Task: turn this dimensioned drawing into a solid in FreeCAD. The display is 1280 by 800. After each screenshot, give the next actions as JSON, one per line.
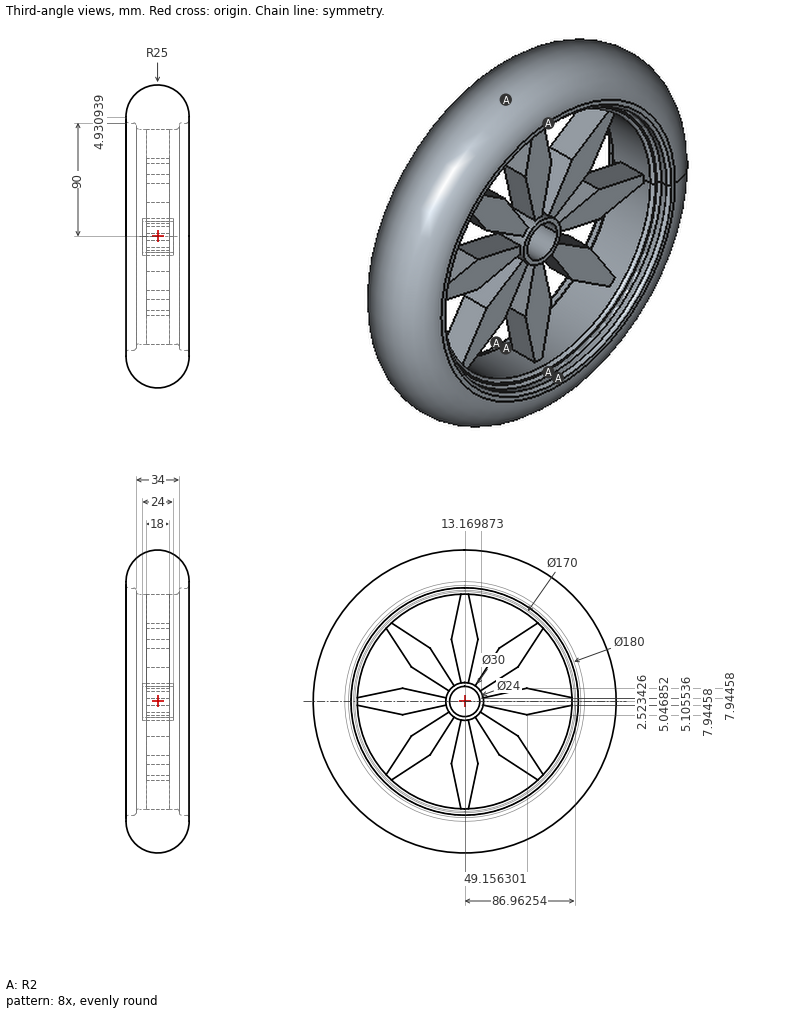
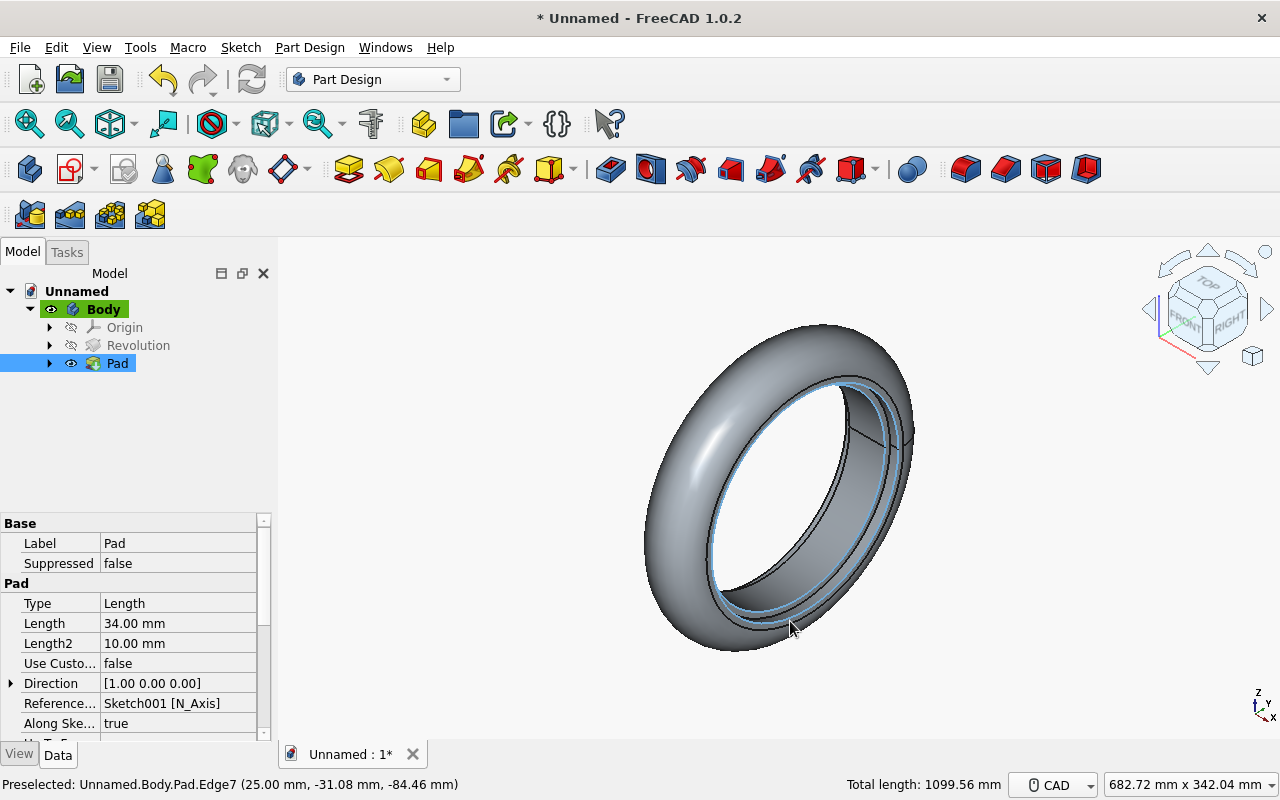
{"action": "key", "text": "2"}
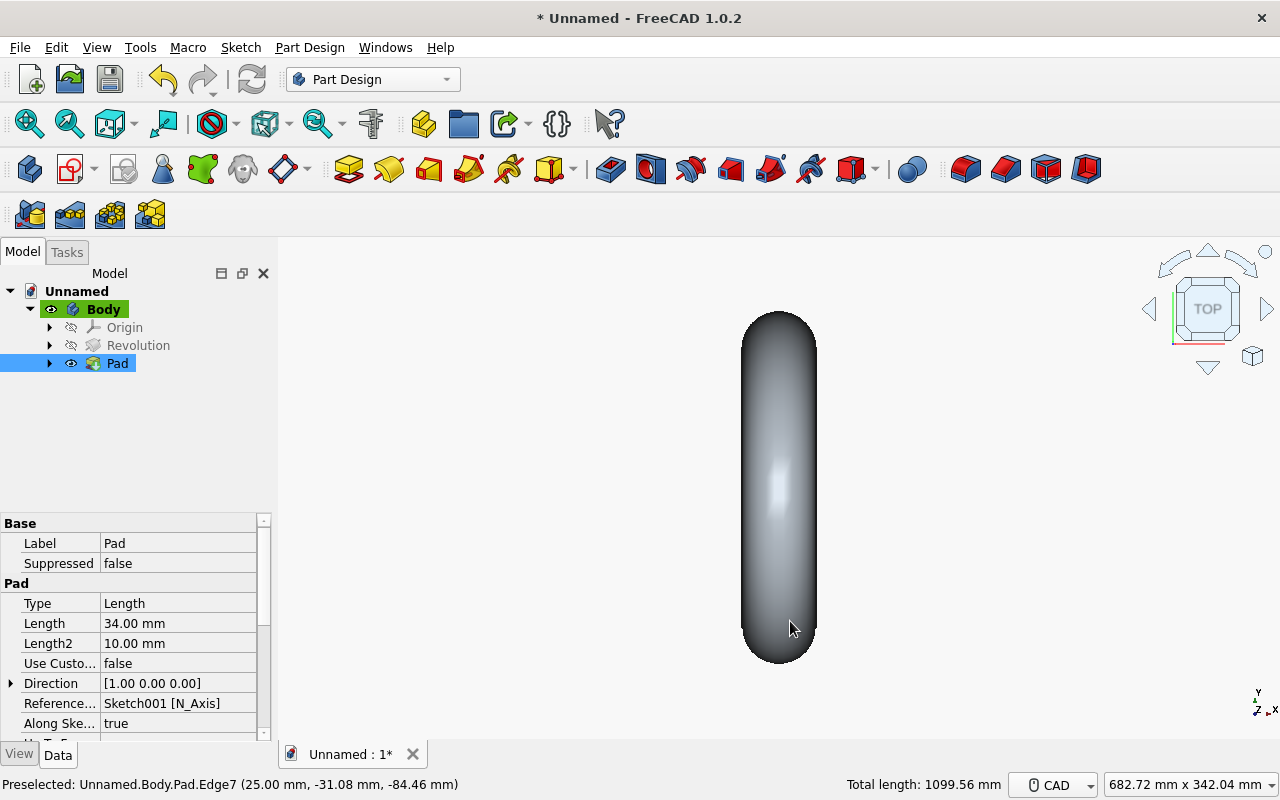
{"action": "key", "text": "1"}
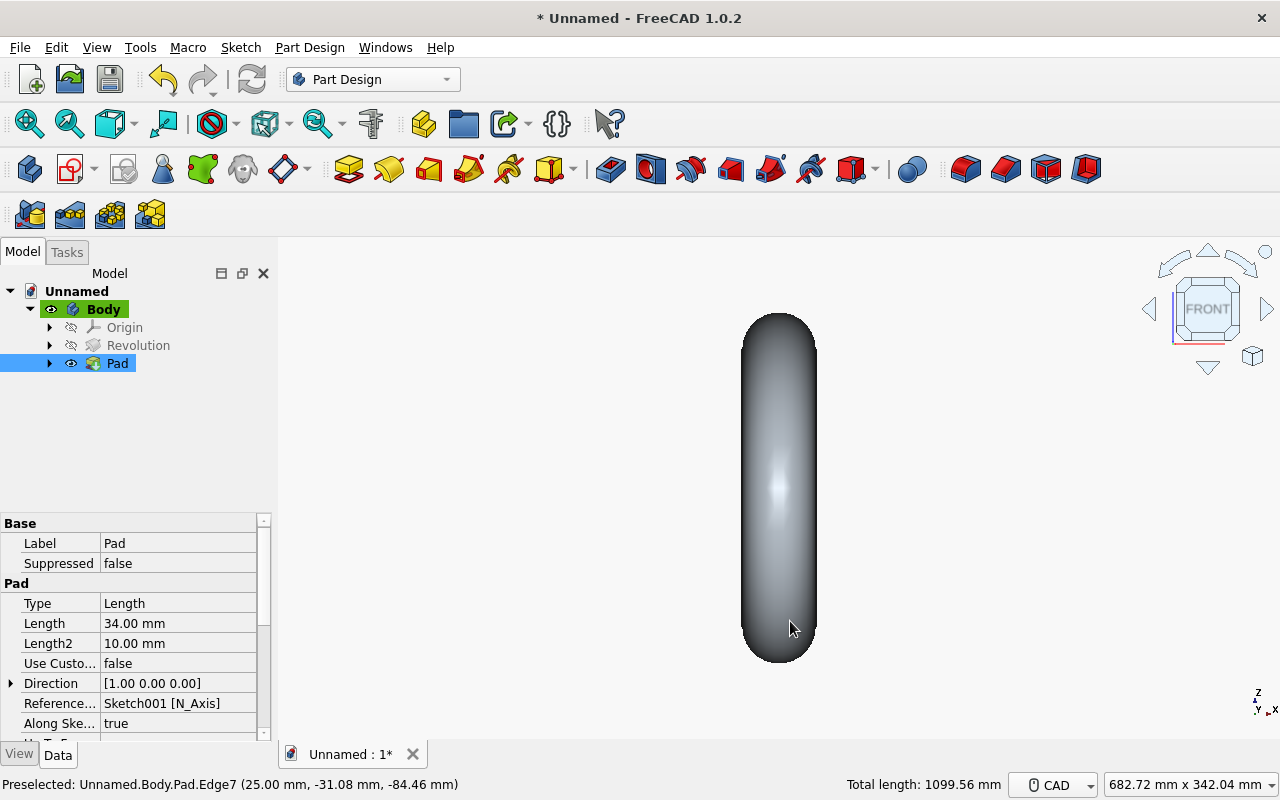
{"action": "key", "text": "3"}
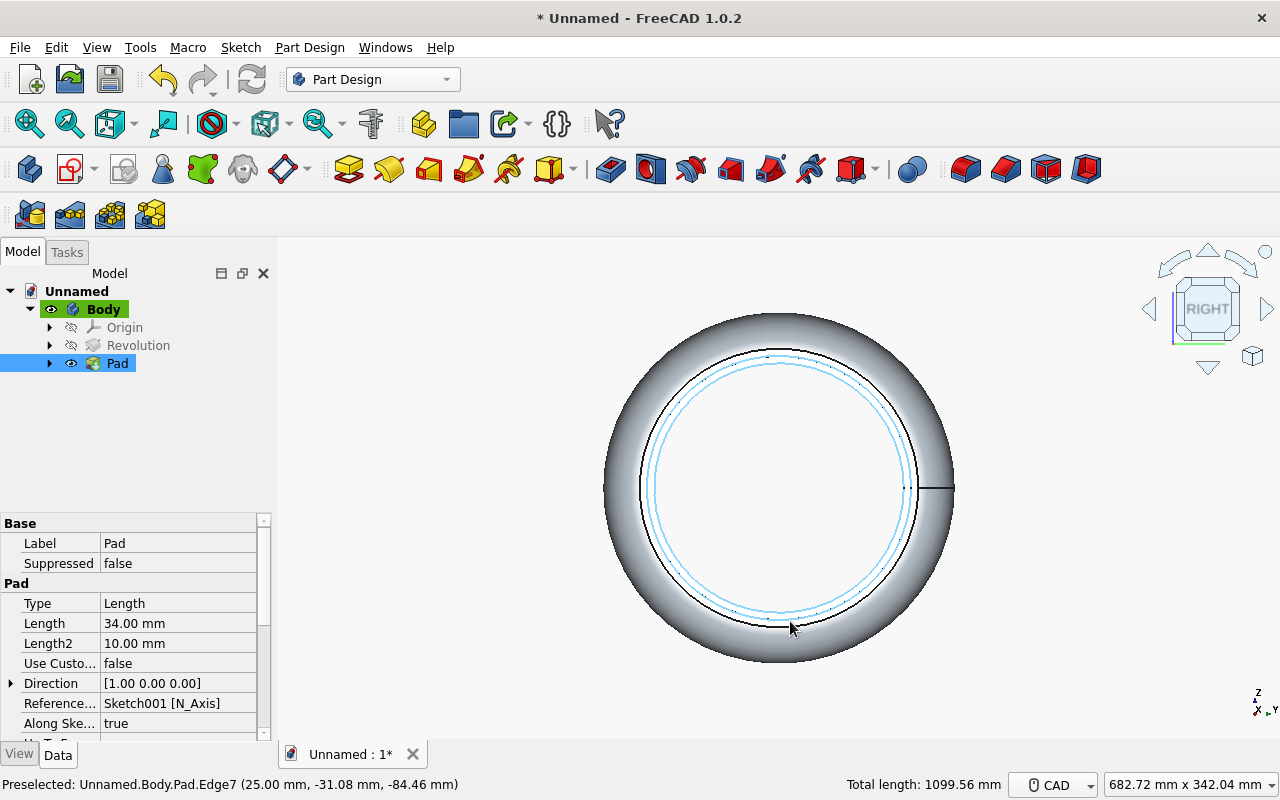
{"action": "key", "text": "5"}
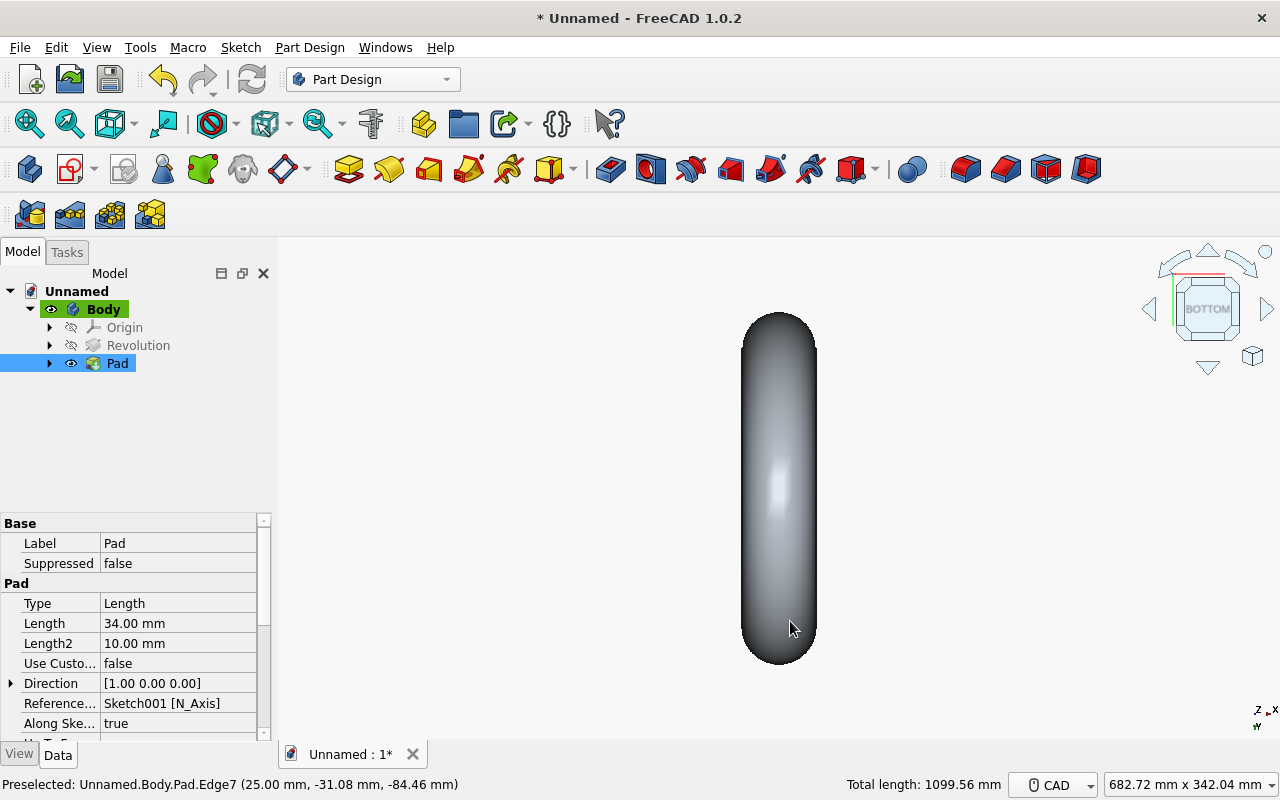
{"action": "key", "text": "4"}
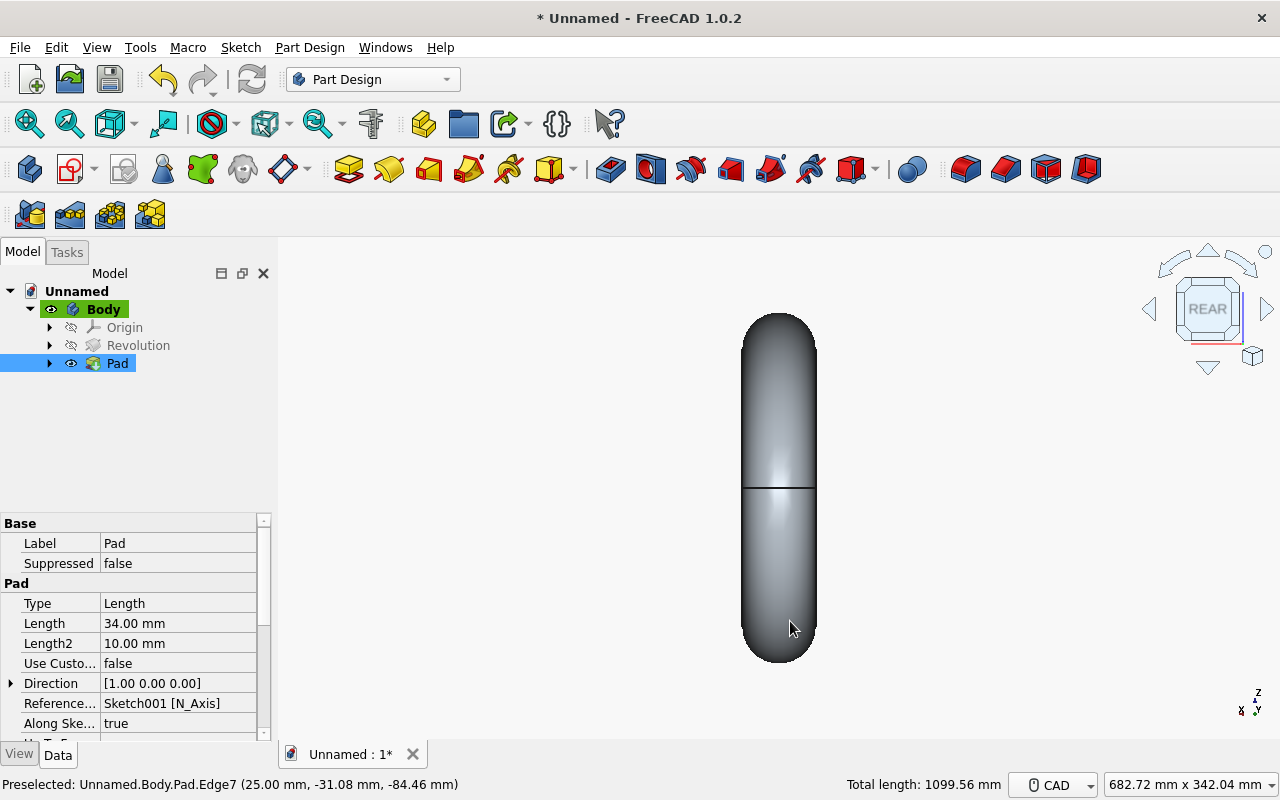
{"action": "key", "text": "6"}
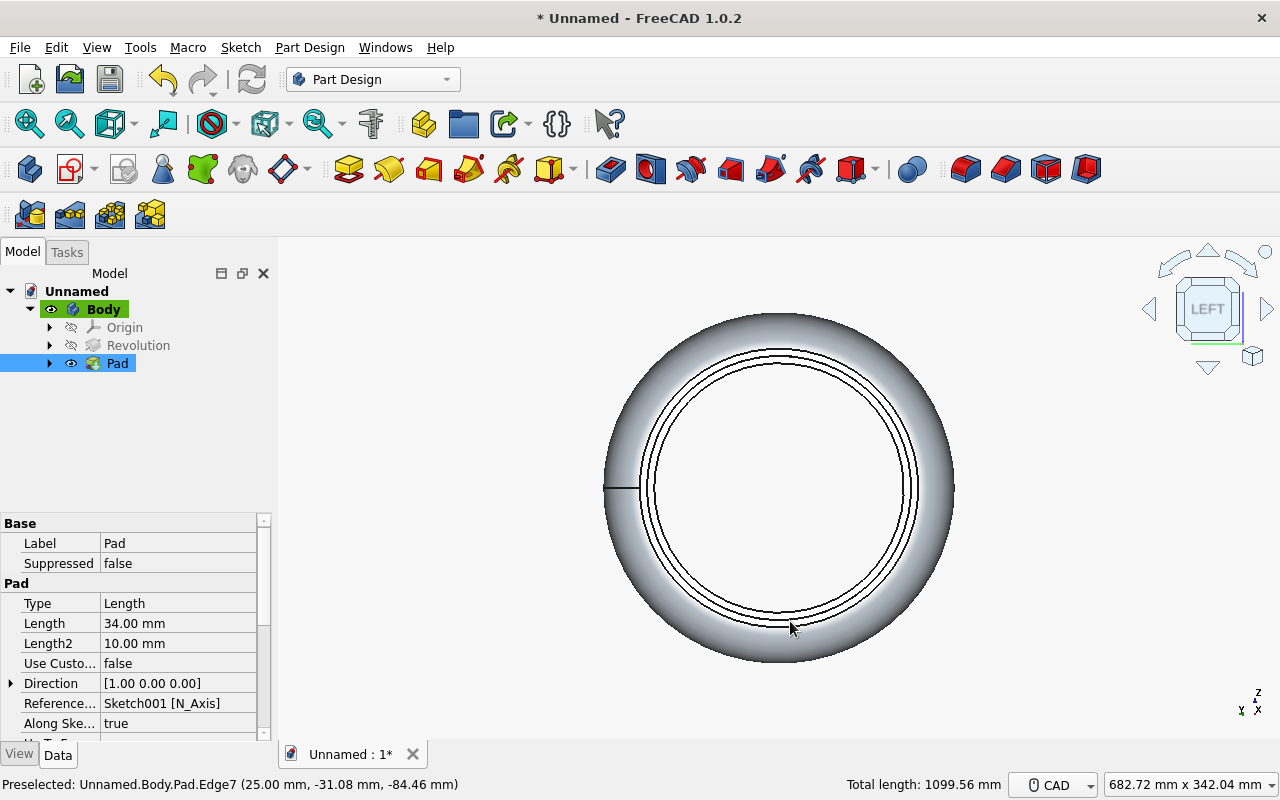
{"action": "left_click", "coordinate": [904, 487], "text": "ctrl"}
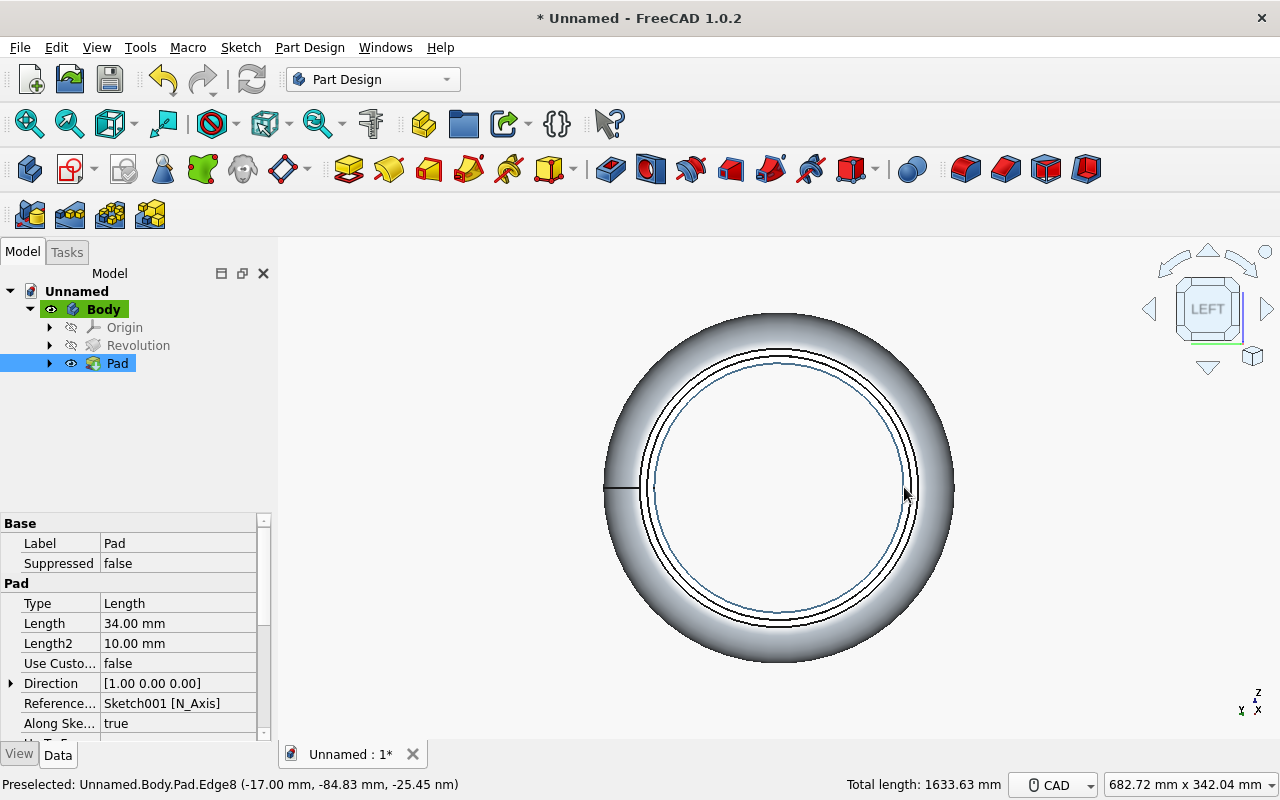
{"action": "left_click", "coordinate": [911, 487], "text": "ctrl"}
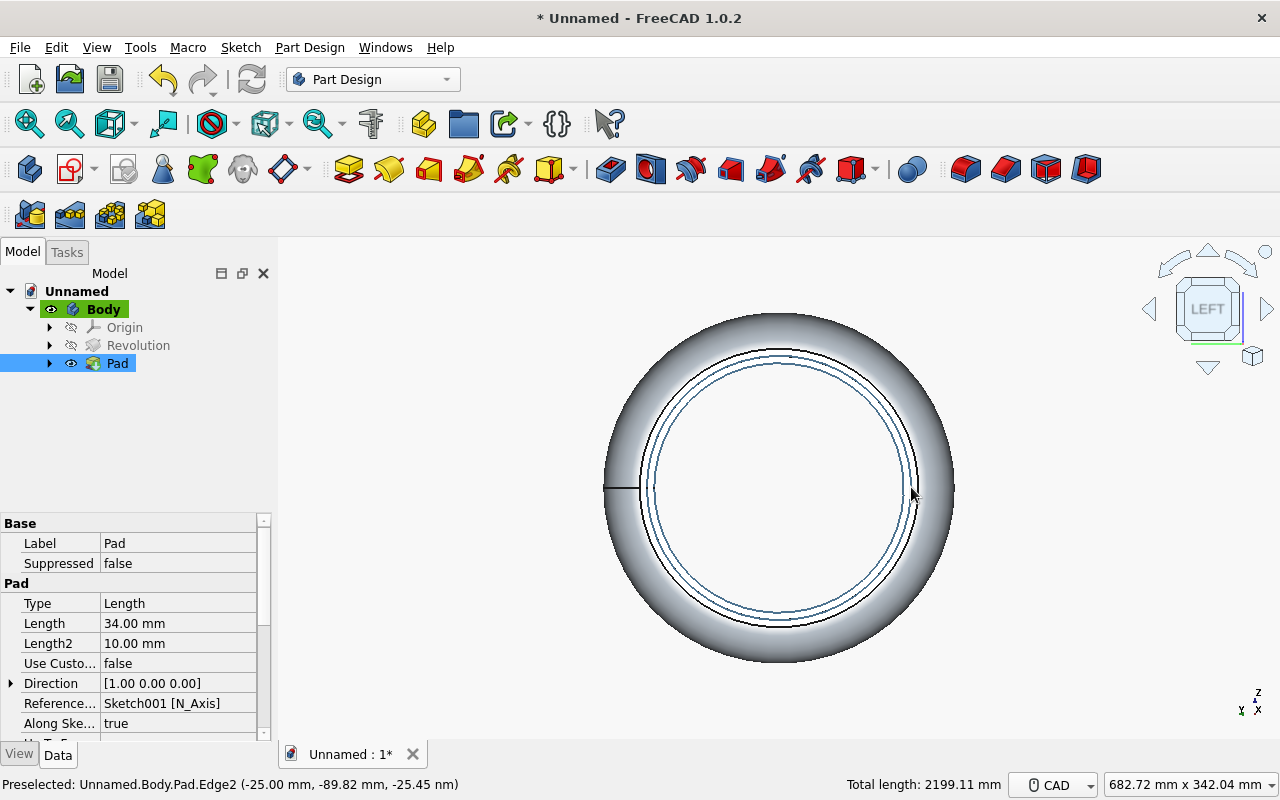
{"action": "key", "text": "v 3"}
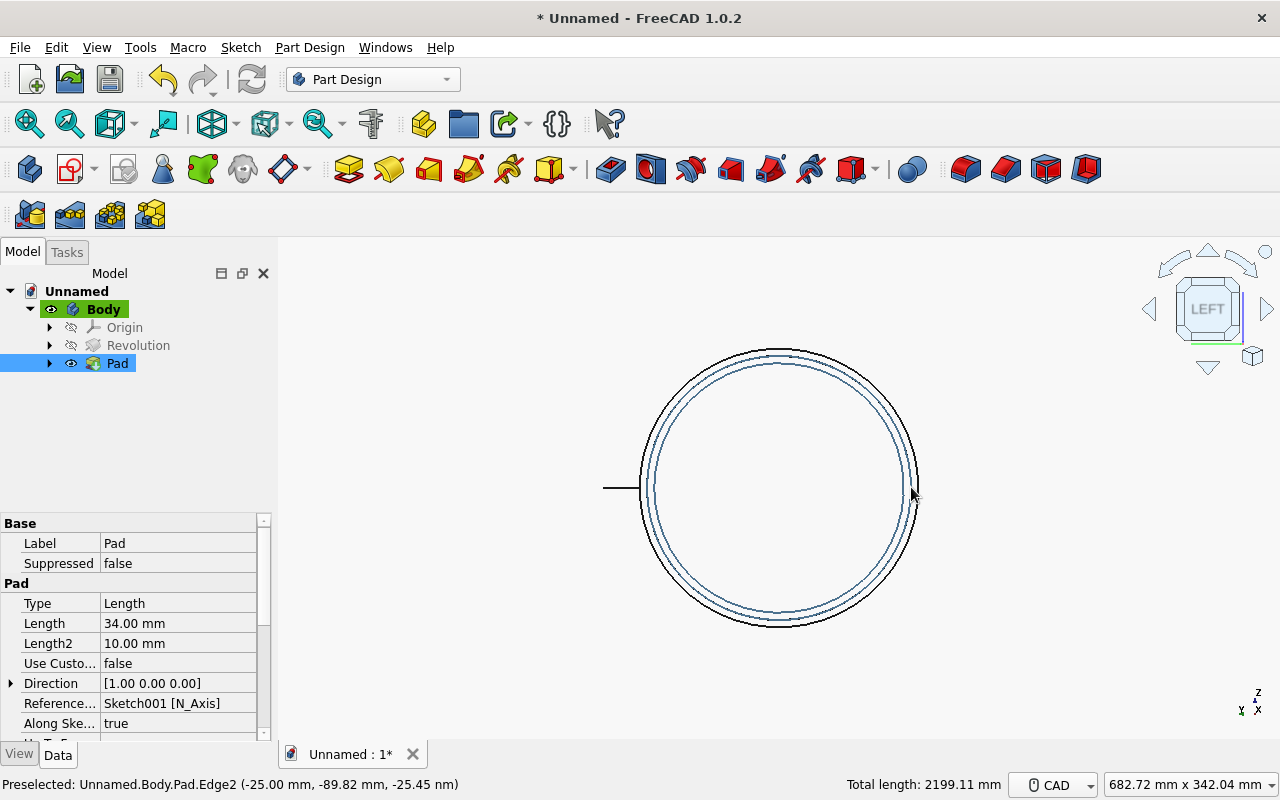
{"action": "key", "text": "0"}